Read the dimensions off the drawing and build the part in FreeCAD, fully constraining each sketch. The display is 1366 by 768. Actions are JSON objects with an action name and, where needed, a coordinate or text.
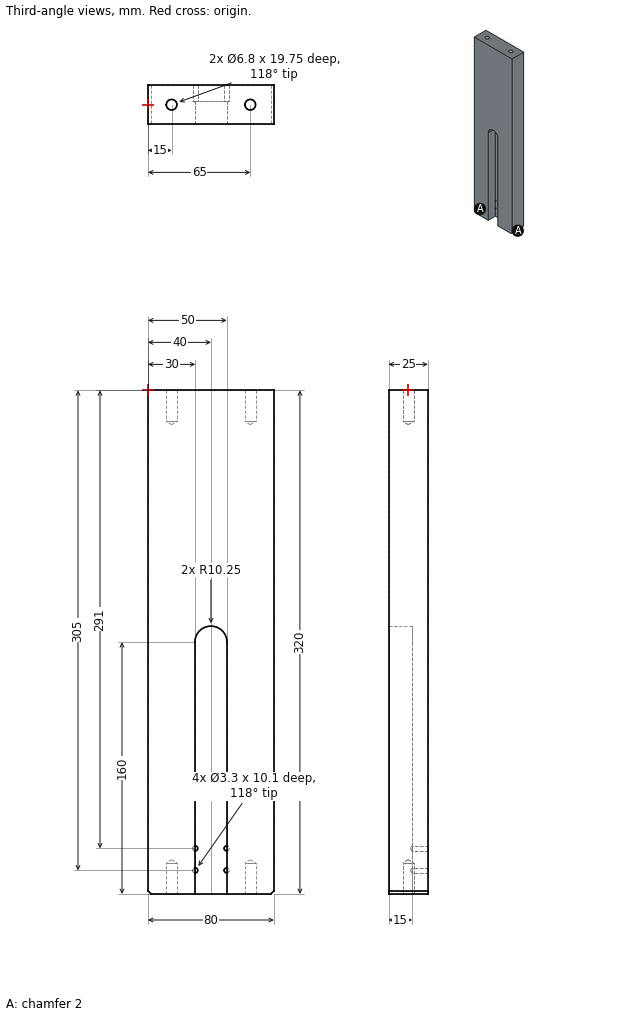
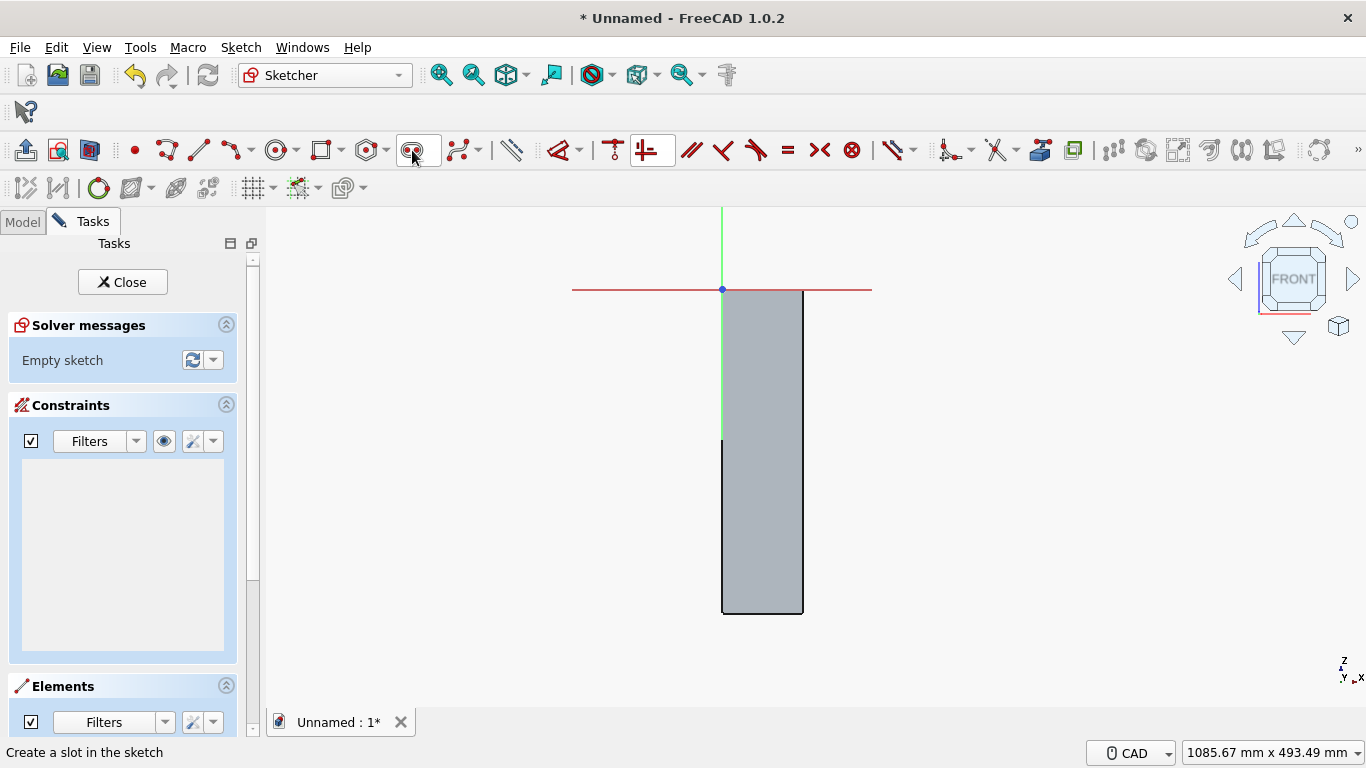
{"action": "scroll", "coordinate": [763, 614], "scroll_direction": "up", "scroll_amount": 4}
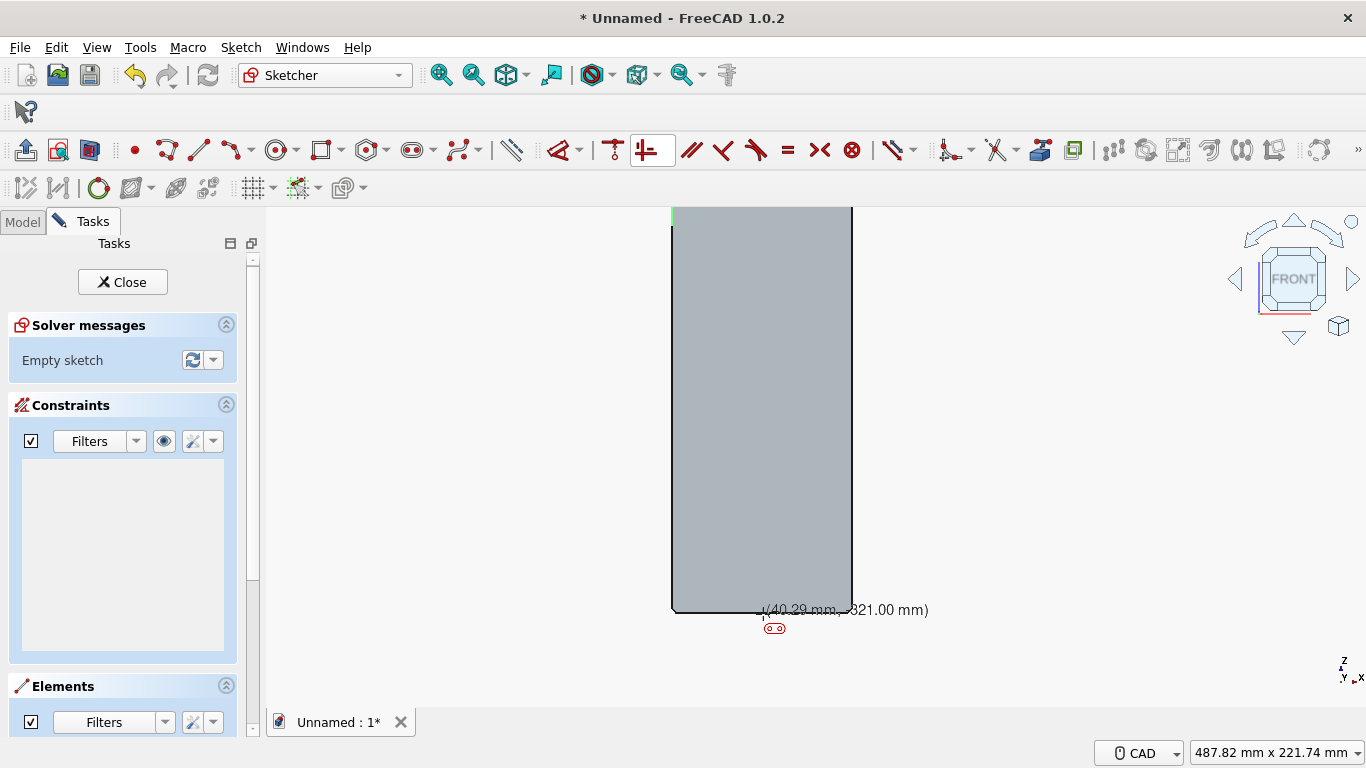
{"action": "left_click", "coordinate": [762, 613]}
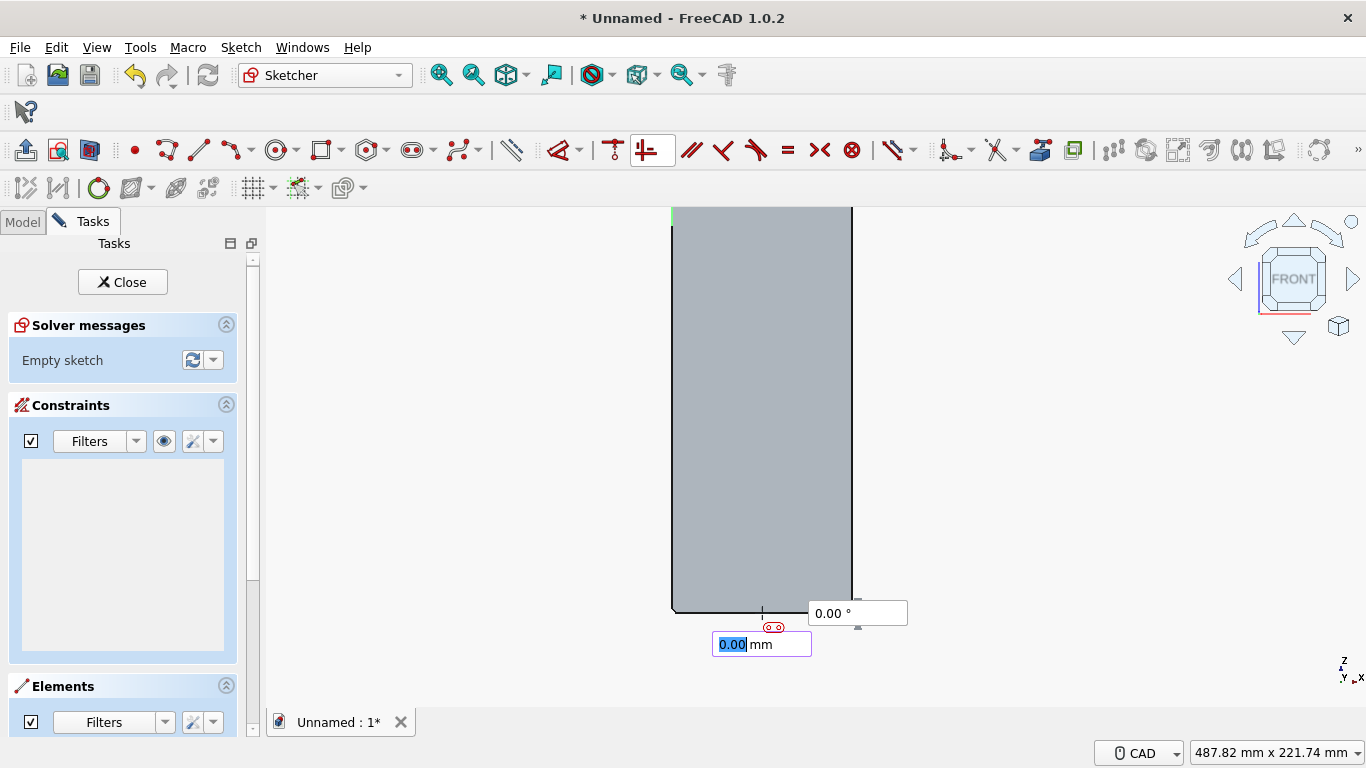
{"action": "left_click", "coordinate": [762, 252]}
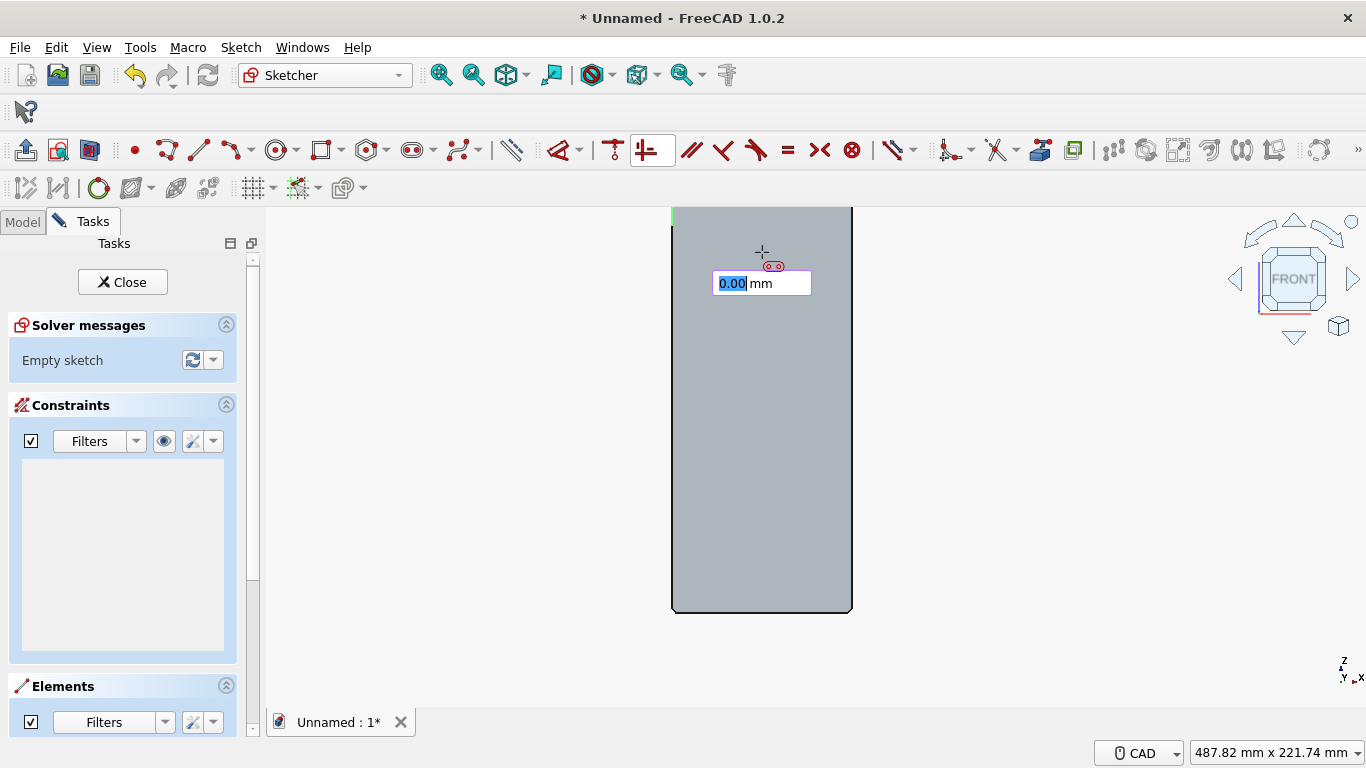
{"action": "left_click", "coordinate": [785, 433]}
{"action": "key", "text": "Escape"}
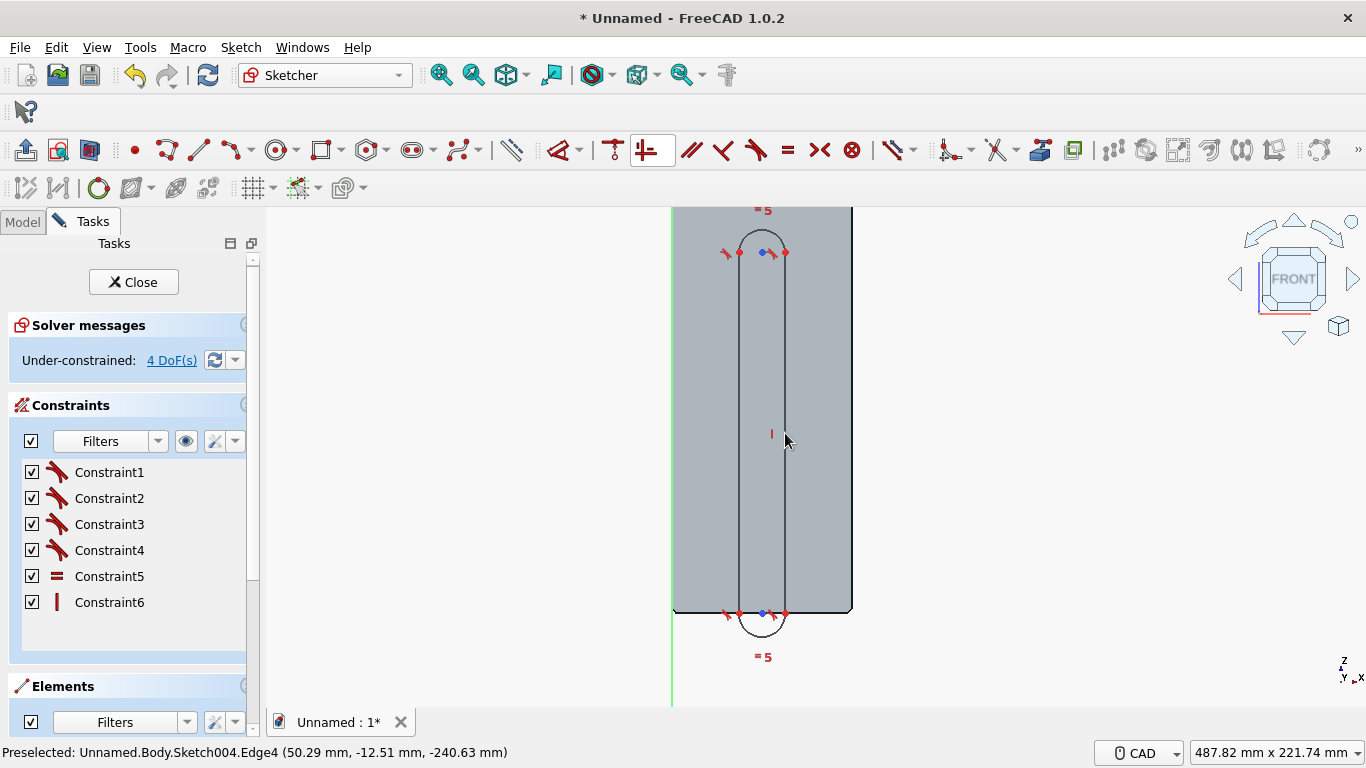
{"action": "left_click", "coordinate": [558, 150]}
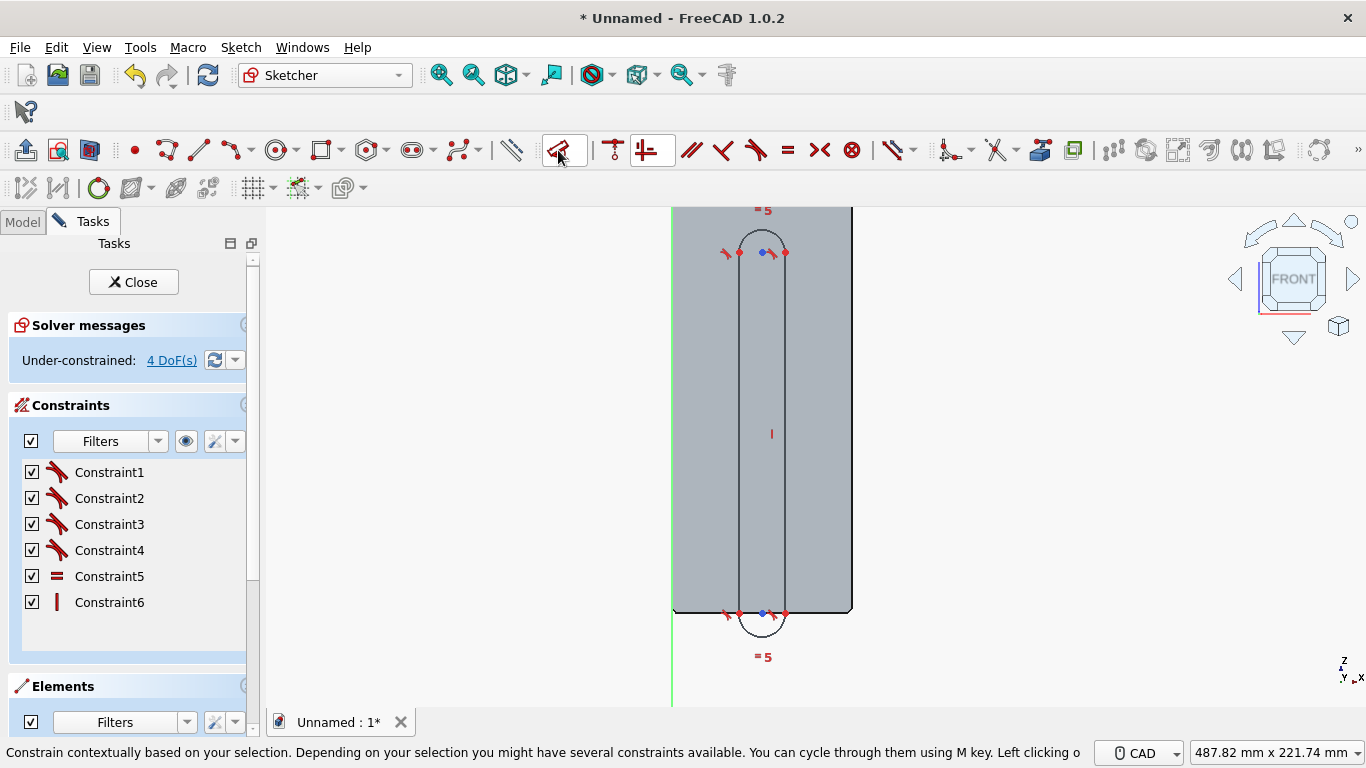
{"action": "scroll", "coordinate": [748, 633], "scroll_direction": "up", "scroll_amount": 3}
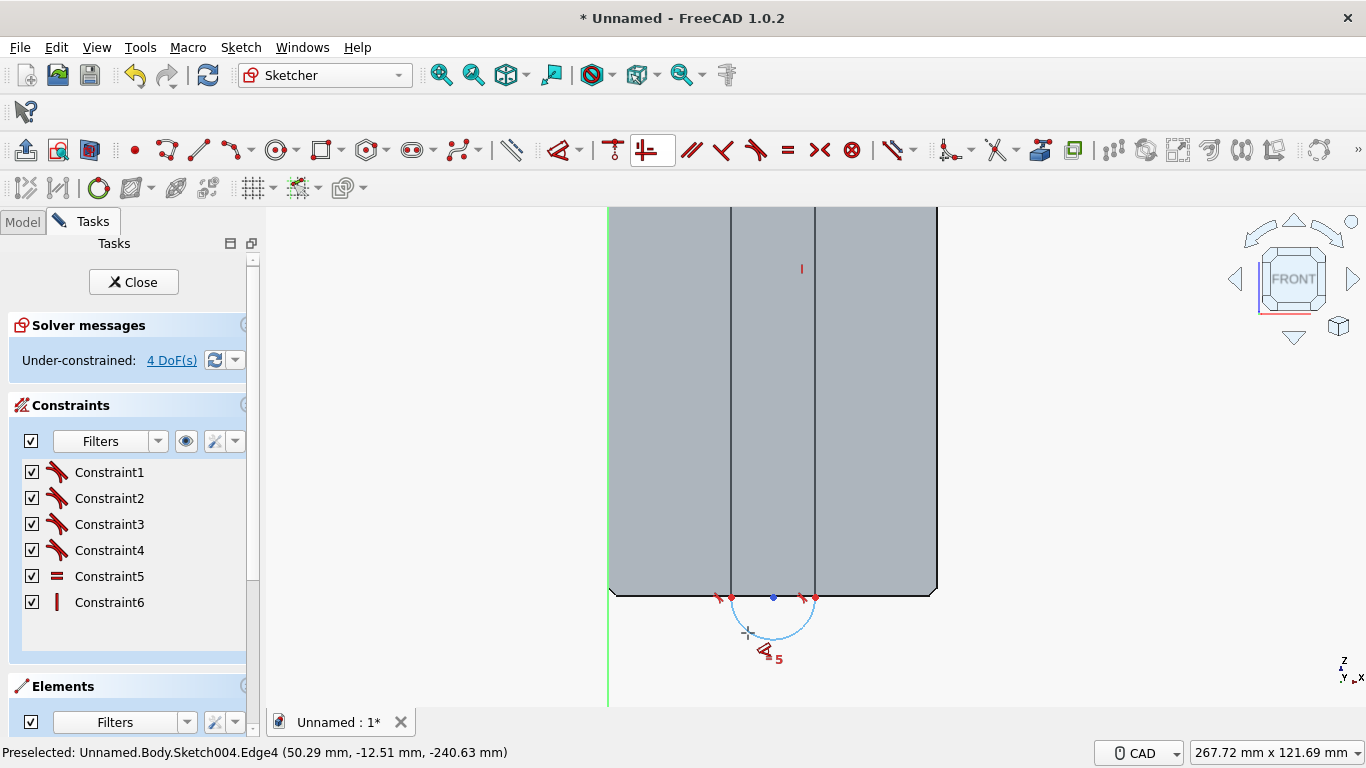
{"action": "left_click", "coordinate": [749, 632]}
{"action": "left_click", "coordinate": [731, 658]}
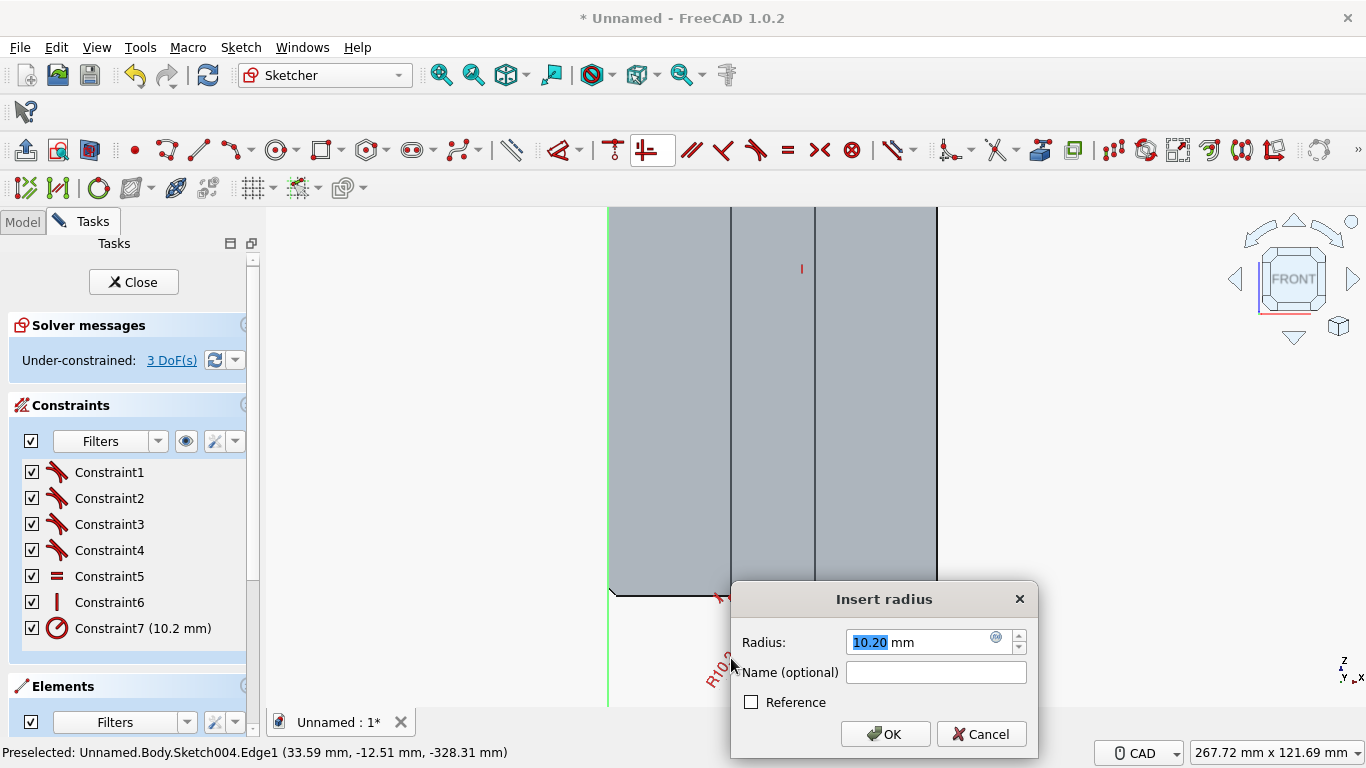
{"action": "type", "text": "10.25"}
{"action": "key", "text": "Return"}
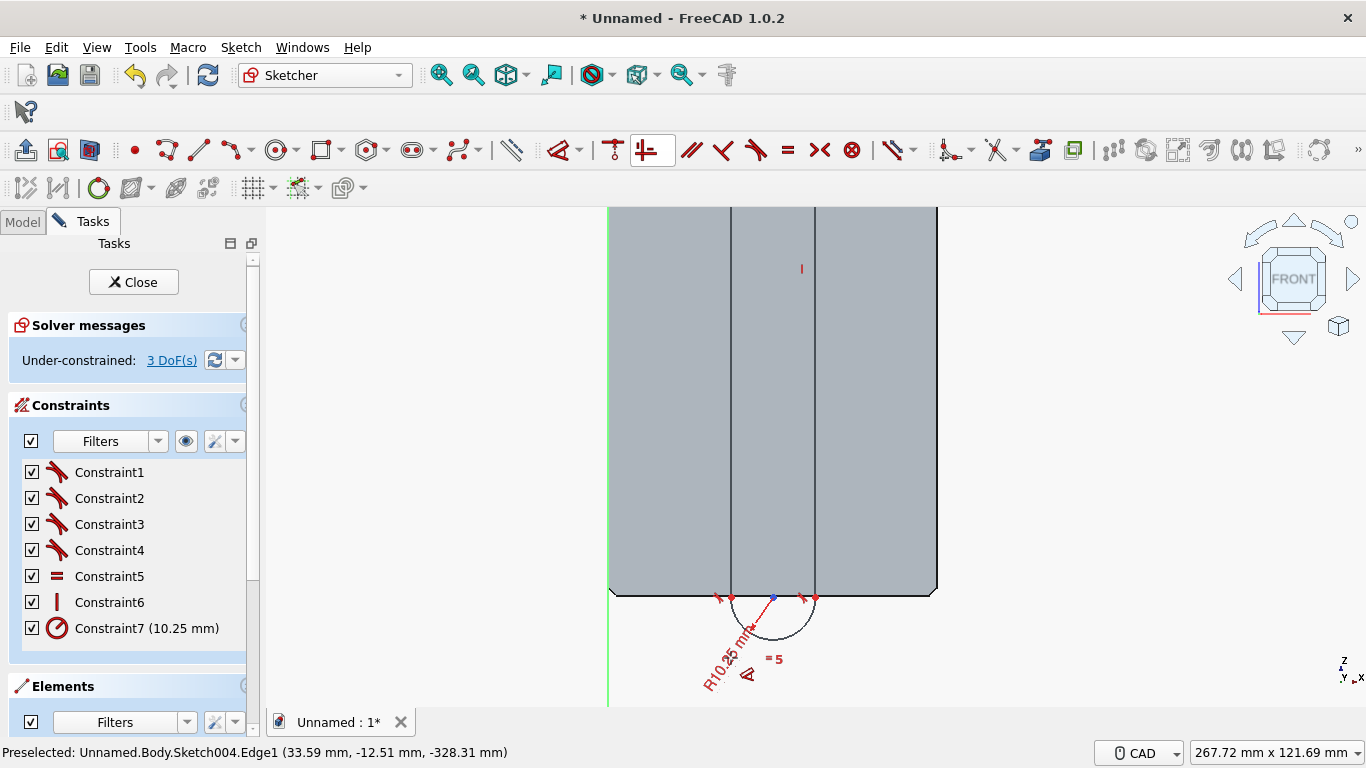
{"action": "scroll", "coordinate": [759, 620], "scroll_direction": "down", "scroll_amount": 7}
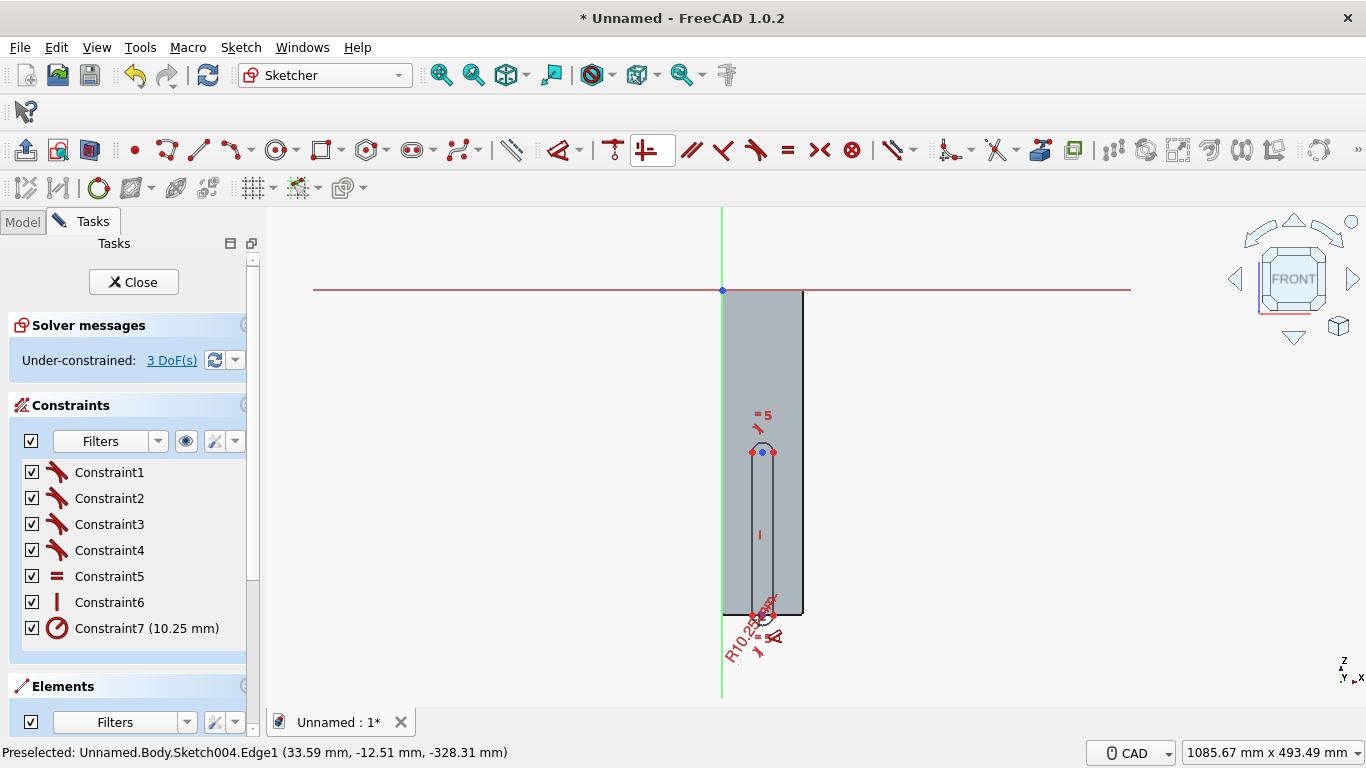
{"action": "left_click", "coordinate": [752, 566]}
{"action": "left_click", "coordinate": [786, 534]}